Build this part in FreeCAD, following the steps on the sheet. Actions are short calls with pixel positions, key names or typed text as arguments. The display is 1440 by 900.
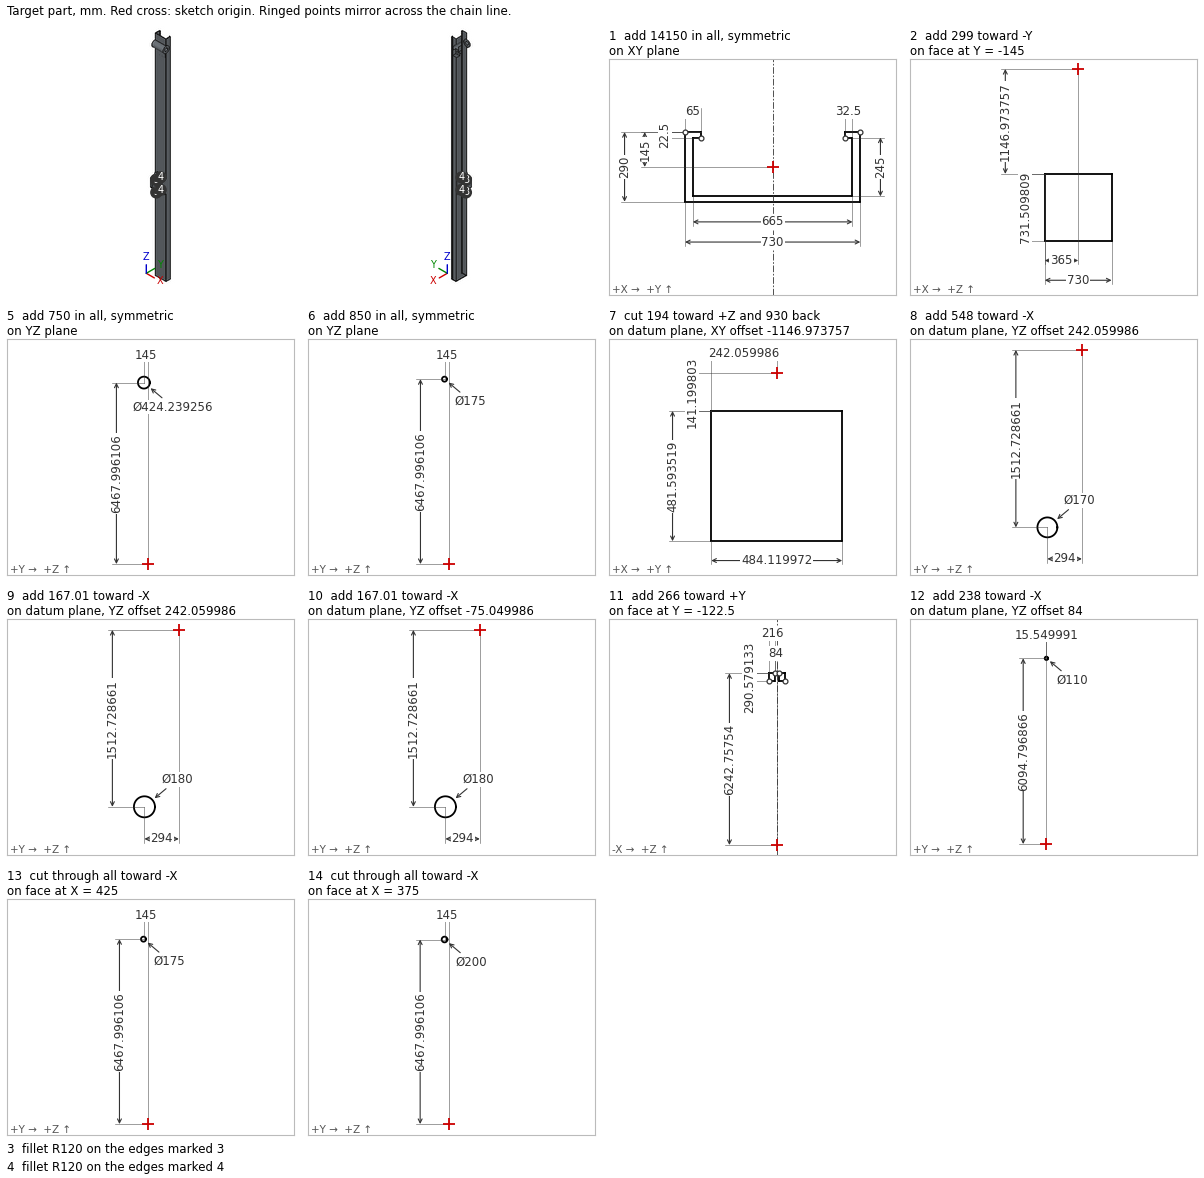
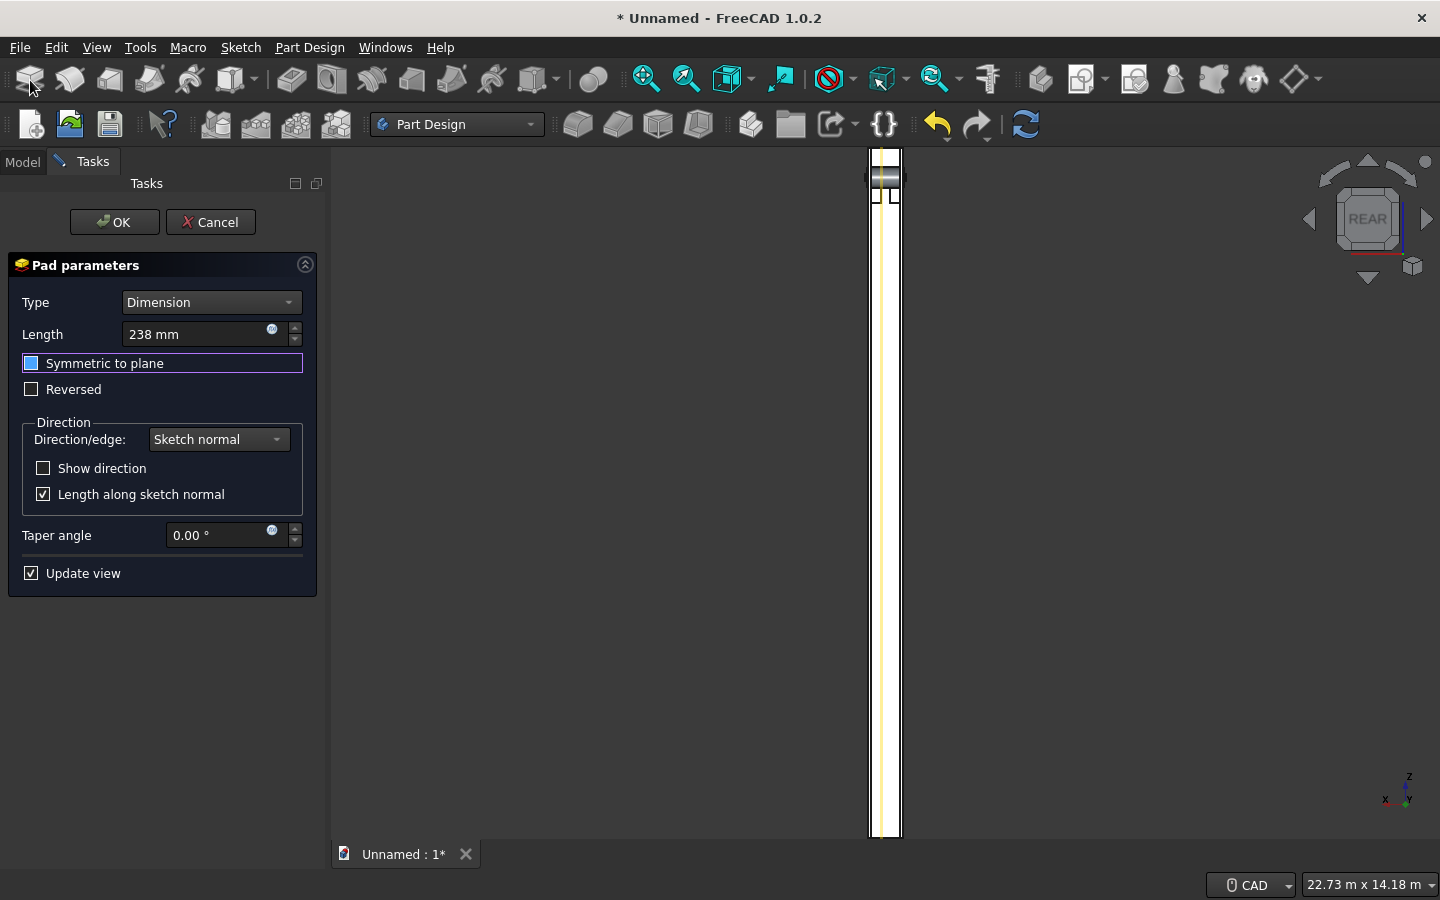
click(30, 389)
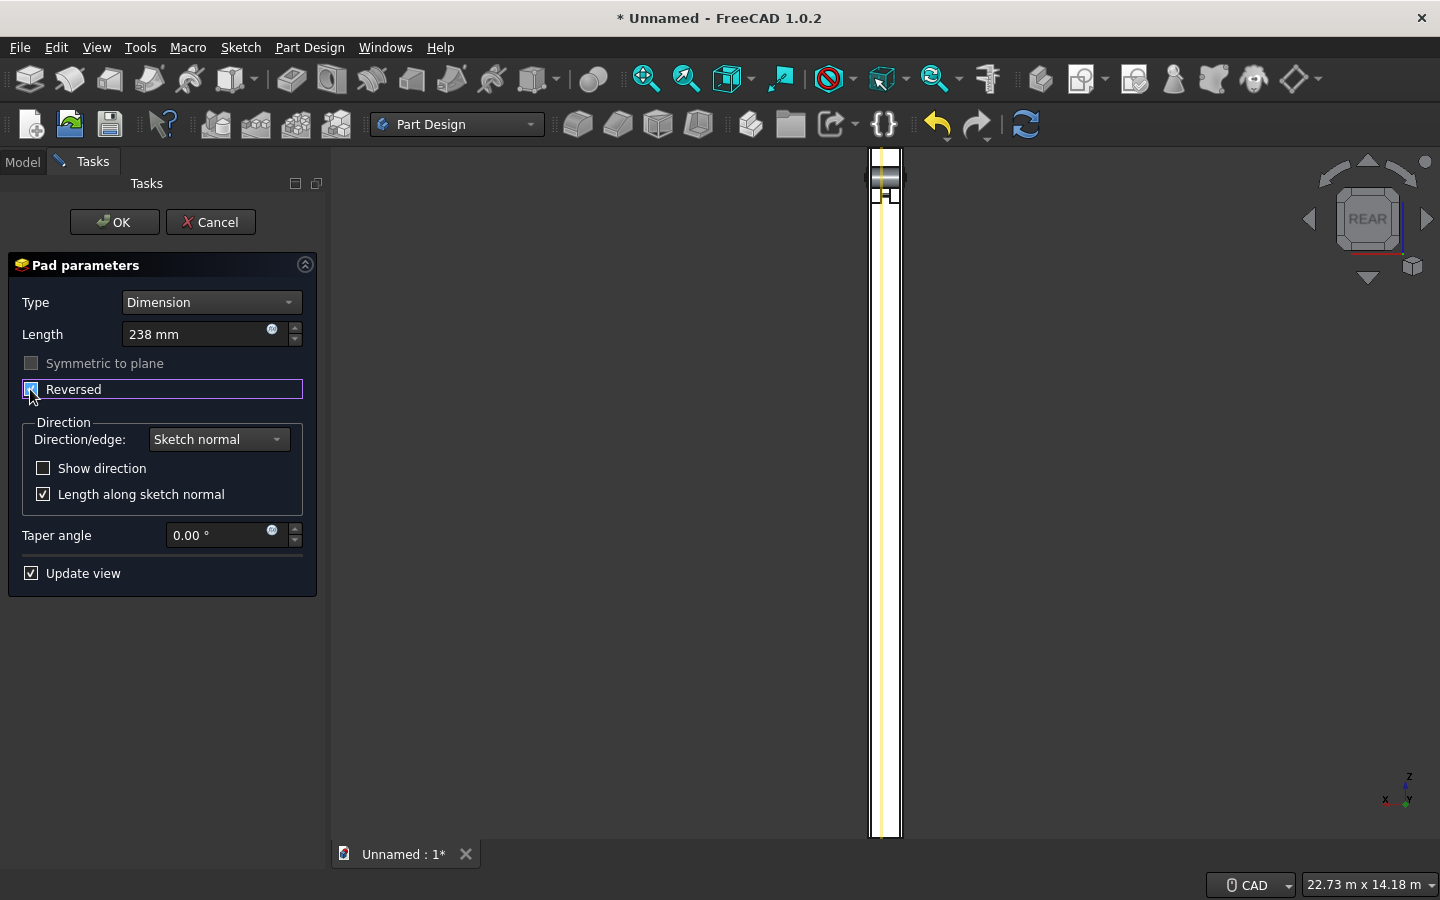
click(115, 222)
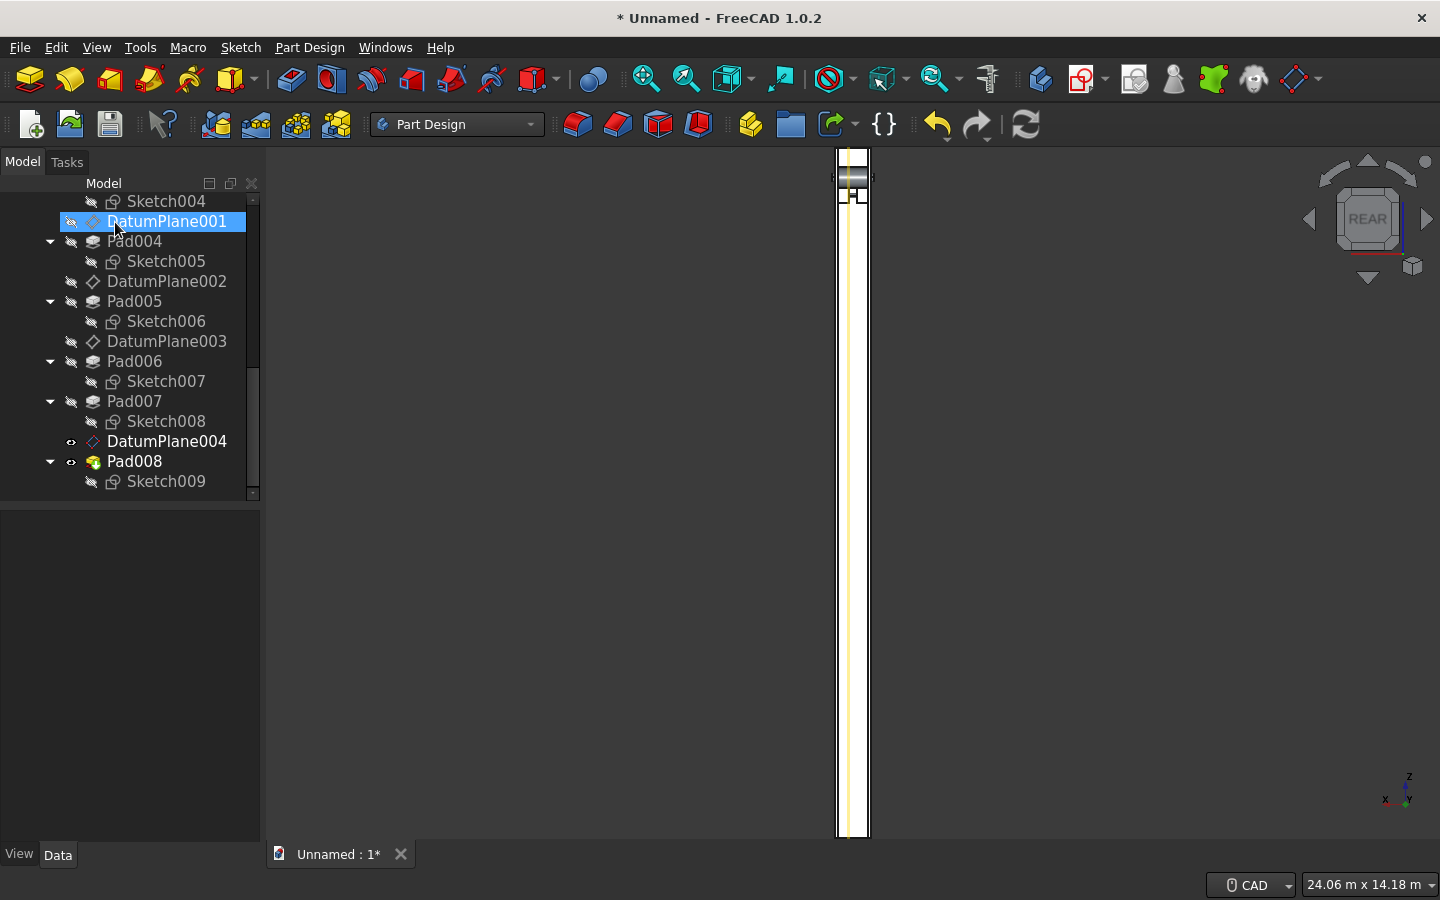
click(116, 442)
key(space)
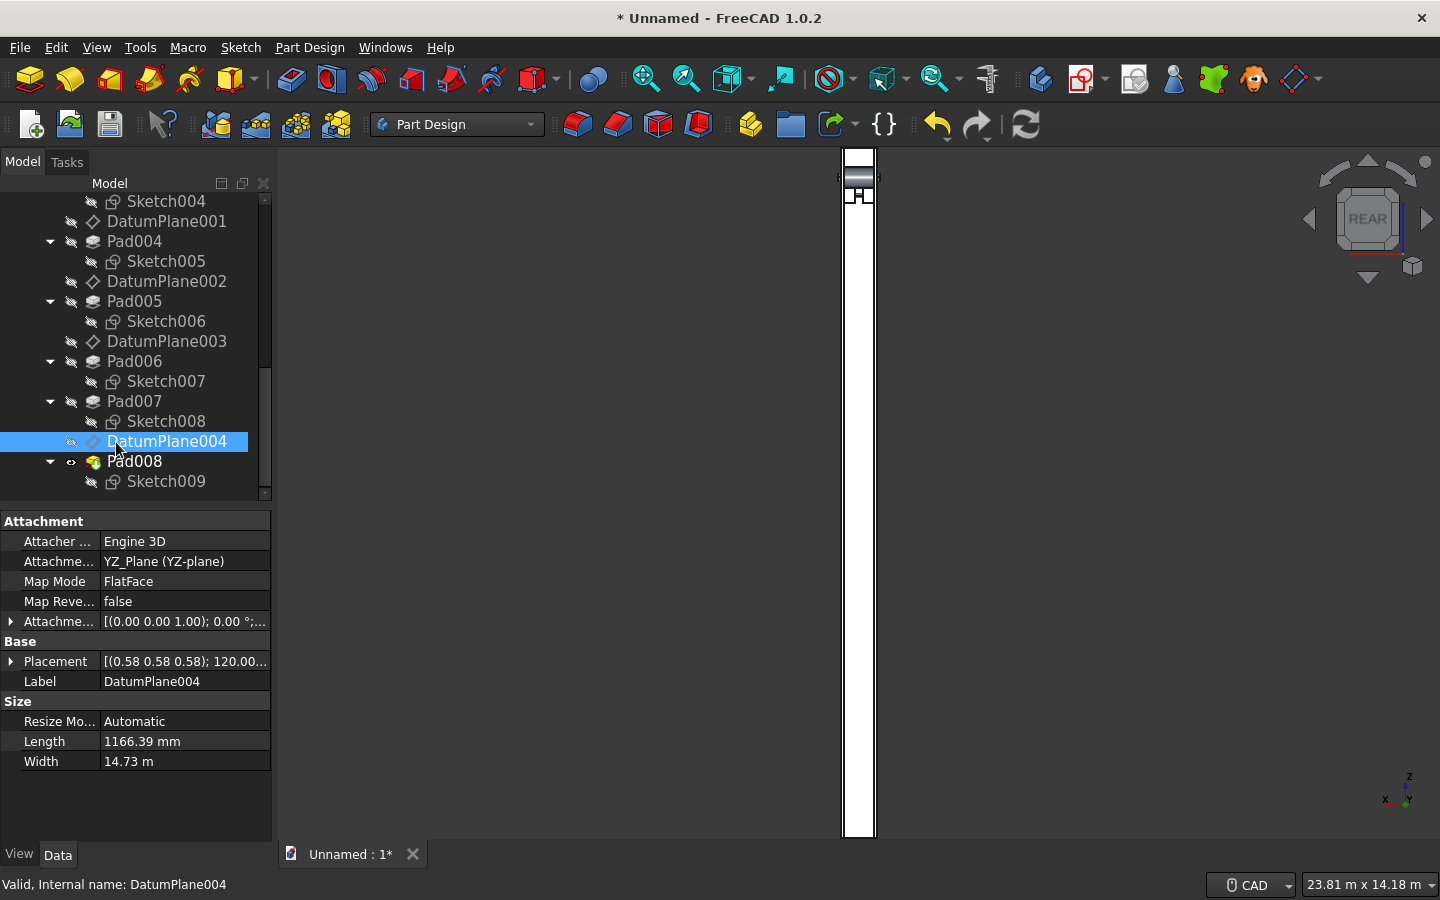
key(0)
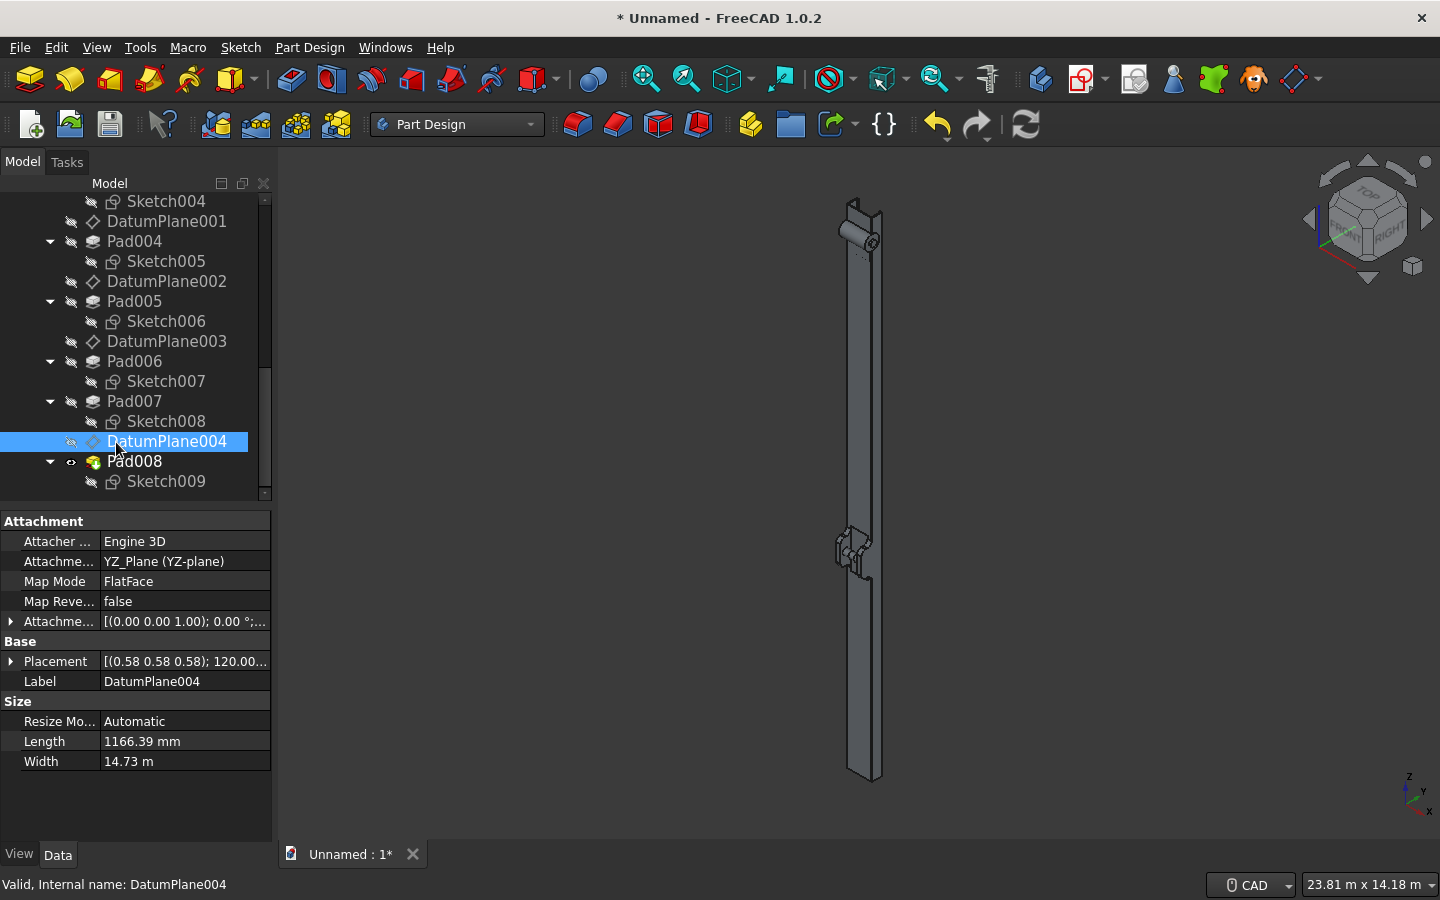
scroll(874, 243, up, 6)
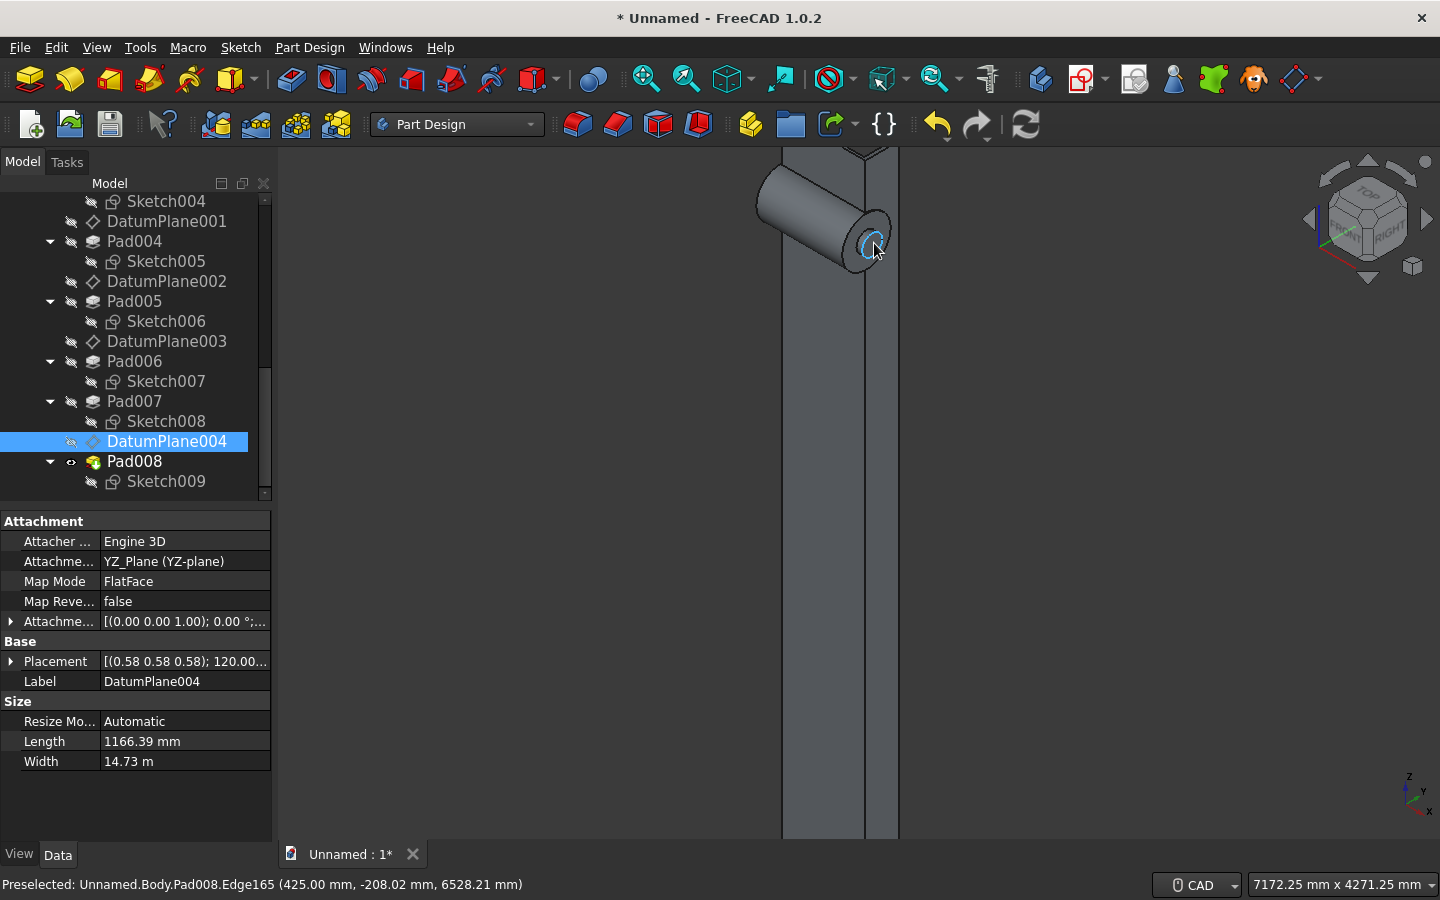
click(875, 242)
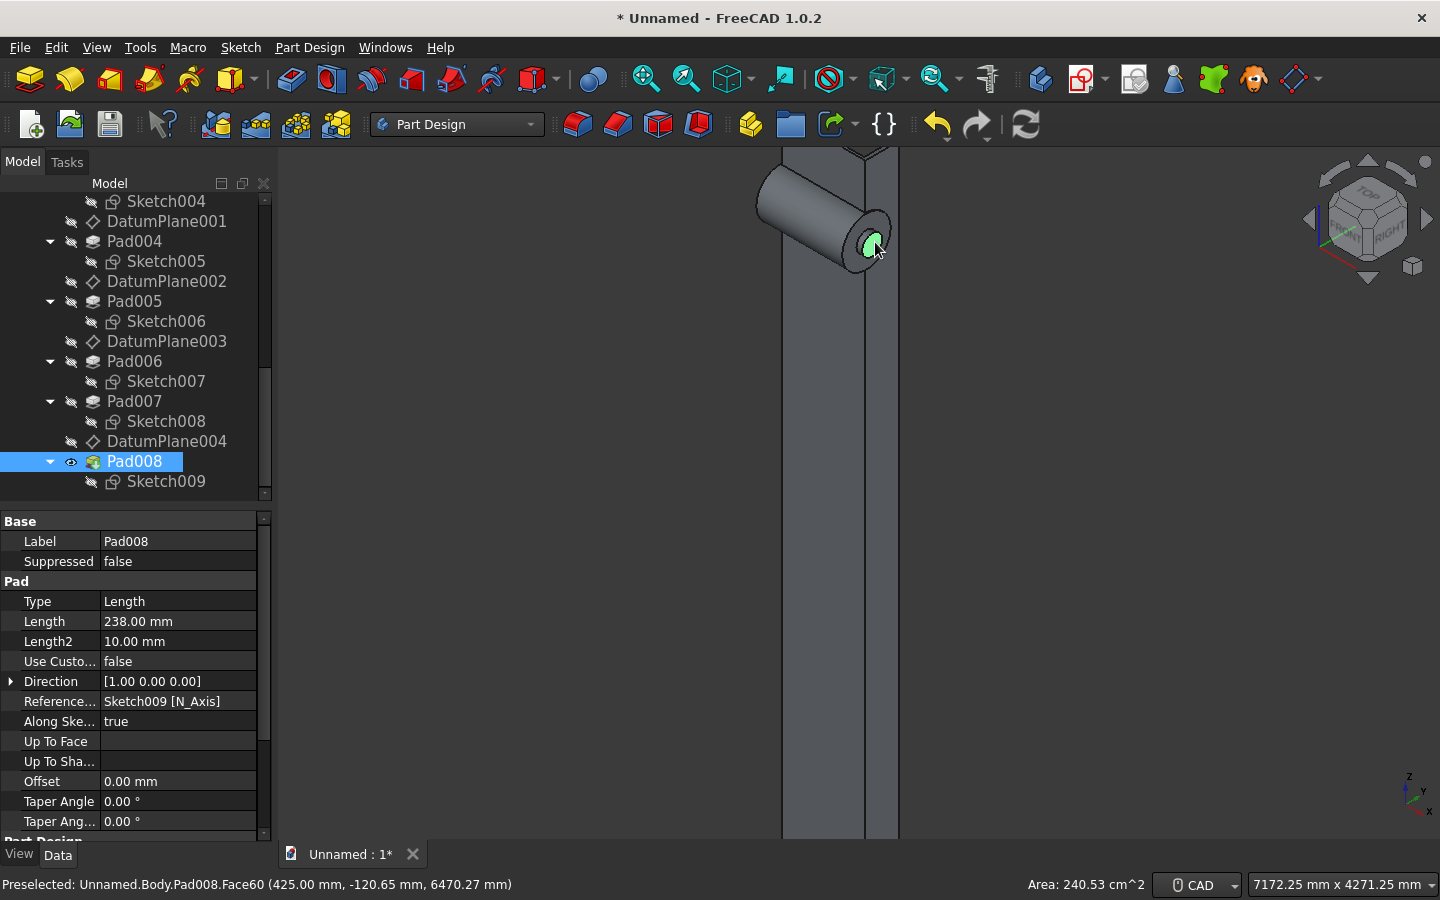
click(1082, 80)